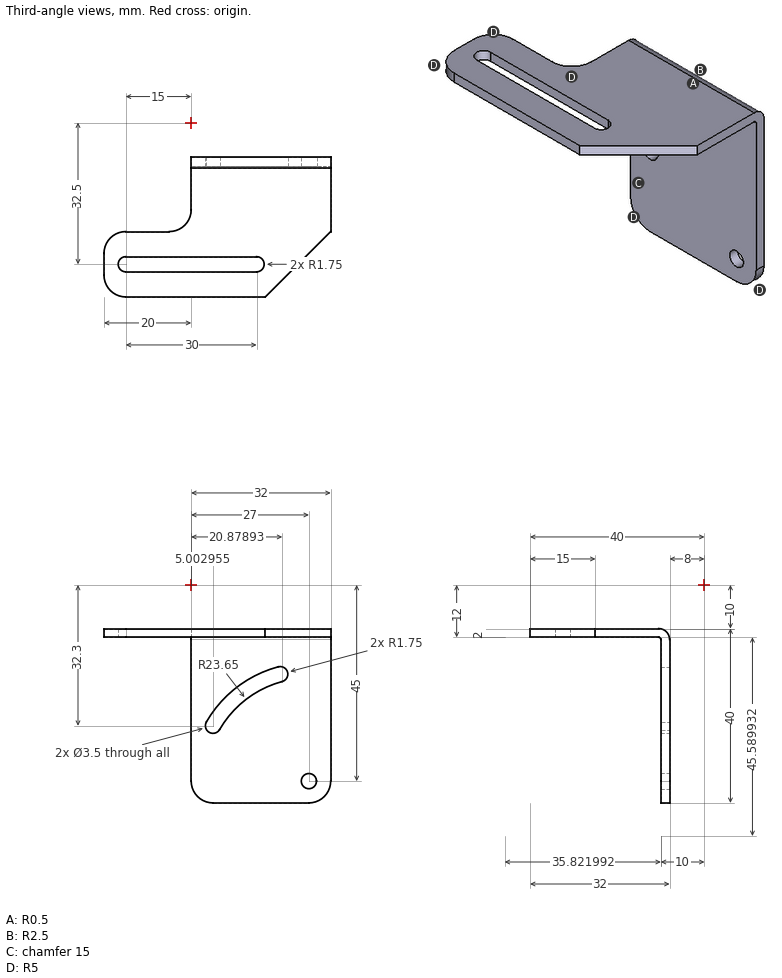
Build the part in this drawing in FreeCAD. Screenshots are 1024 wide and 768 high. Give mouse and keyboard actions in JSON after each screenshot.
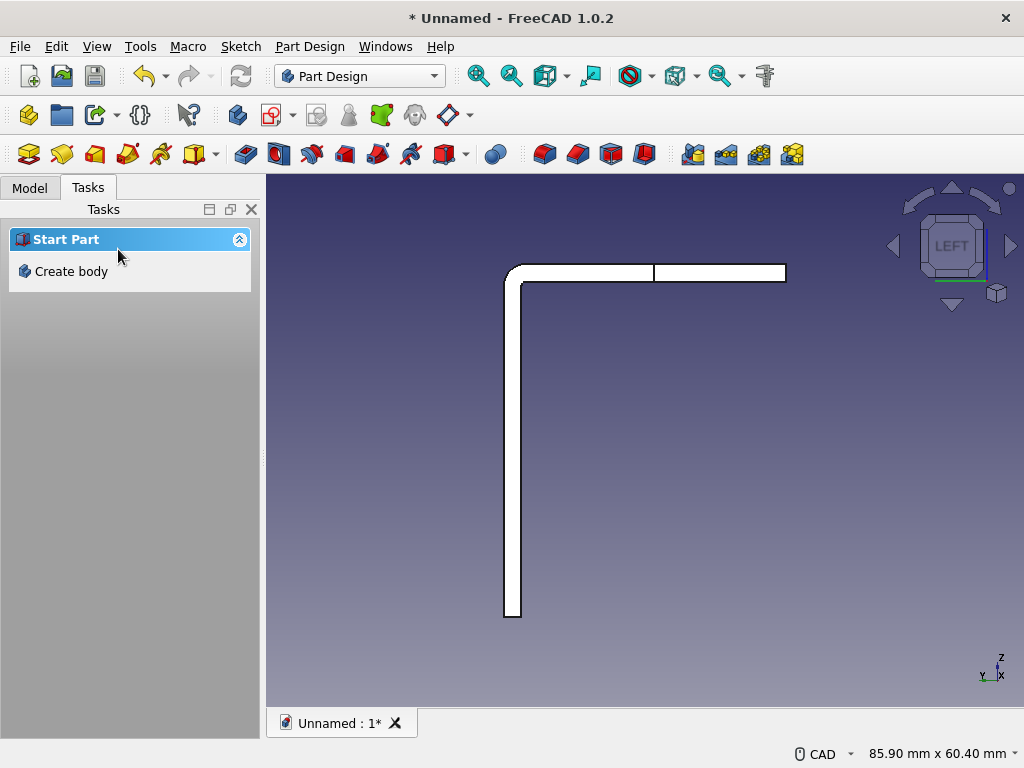
{"action": "key", "text": "5"}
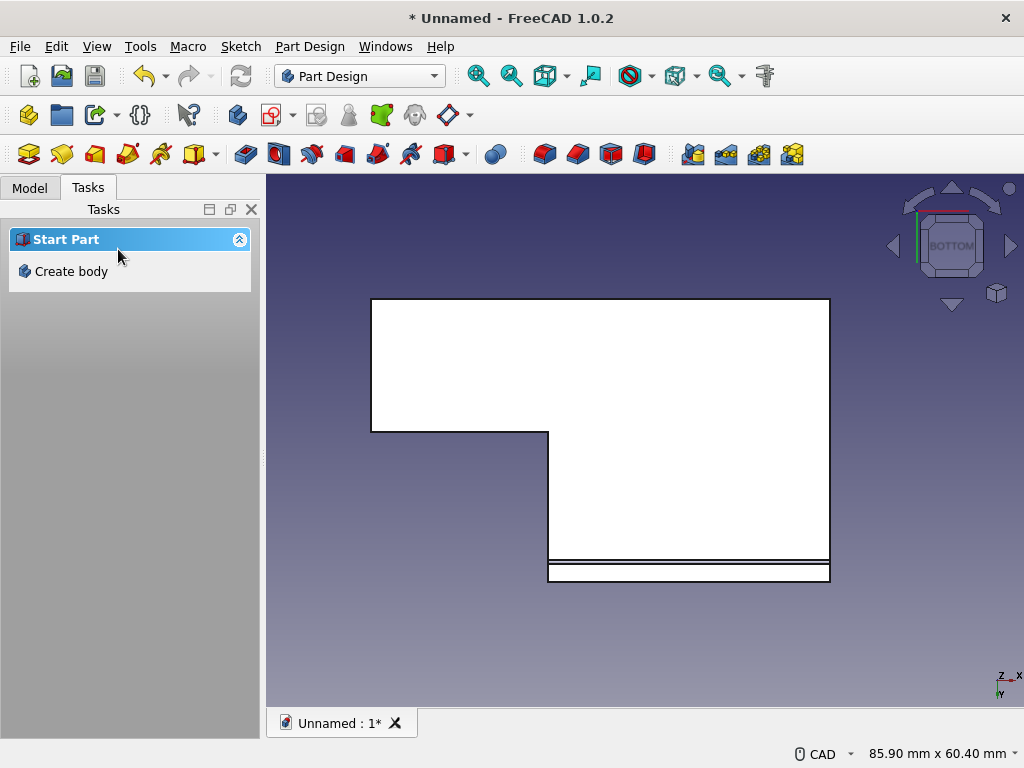
{"action": "left_click", "coordinate": [666, 428]}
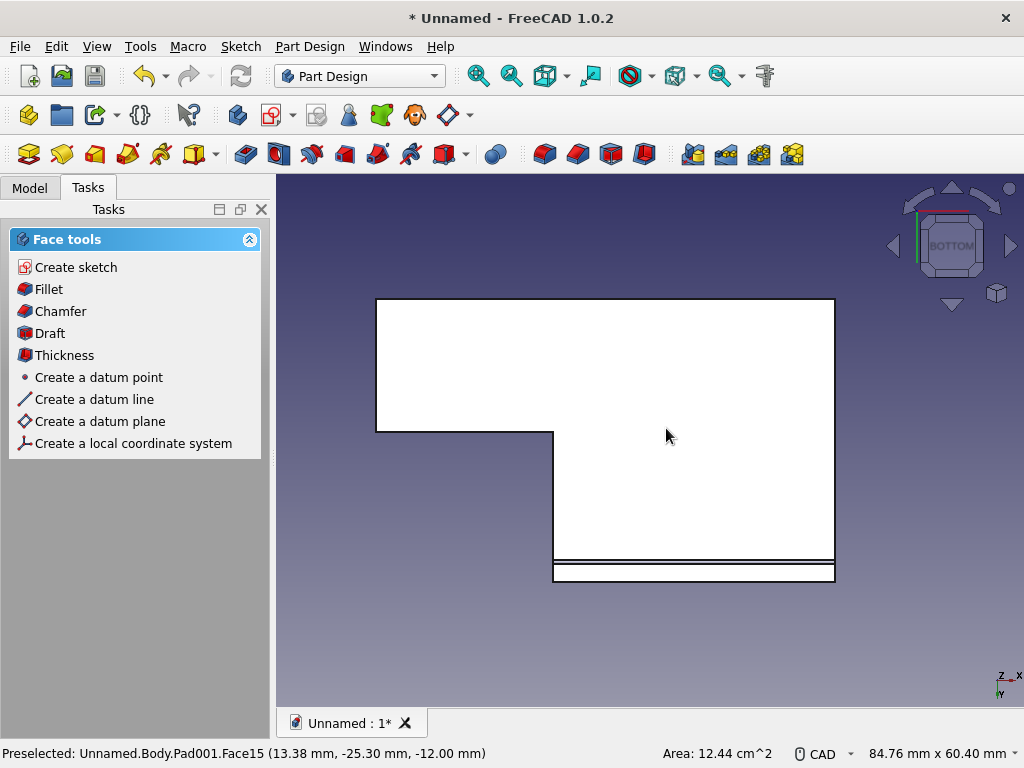
{"action": "left_click", "coordinate": [270, 116]}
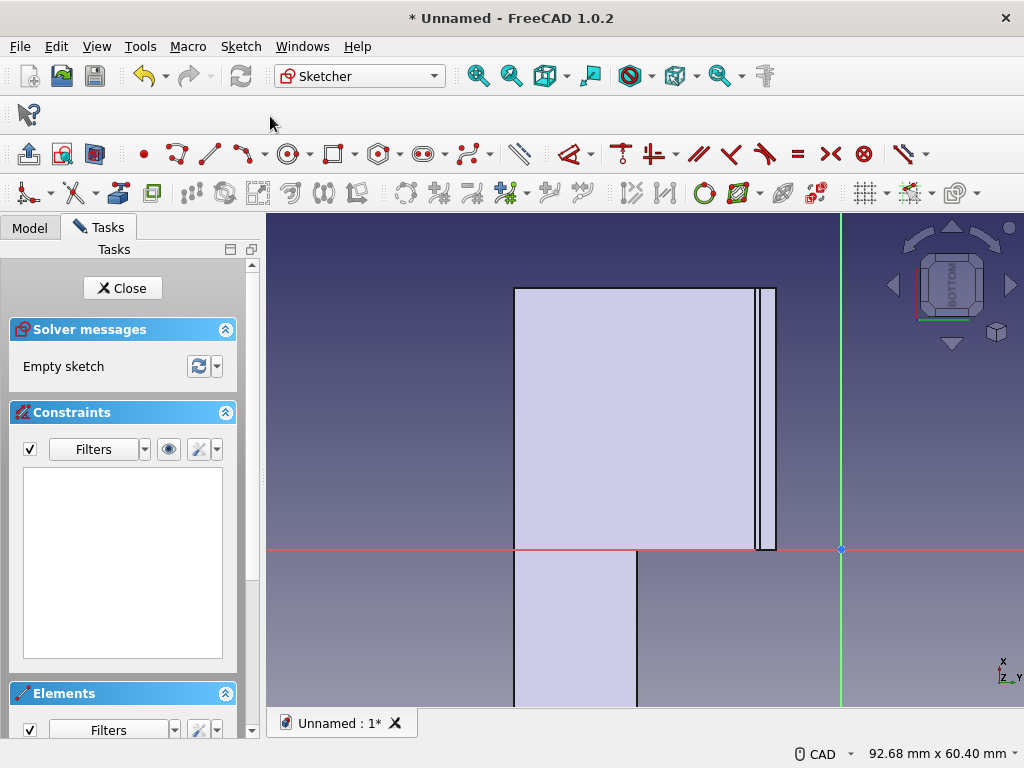
{"action": "scroll", "coordinate": [294, 241], "scroll_direction": "down", "scroll_amount": 1}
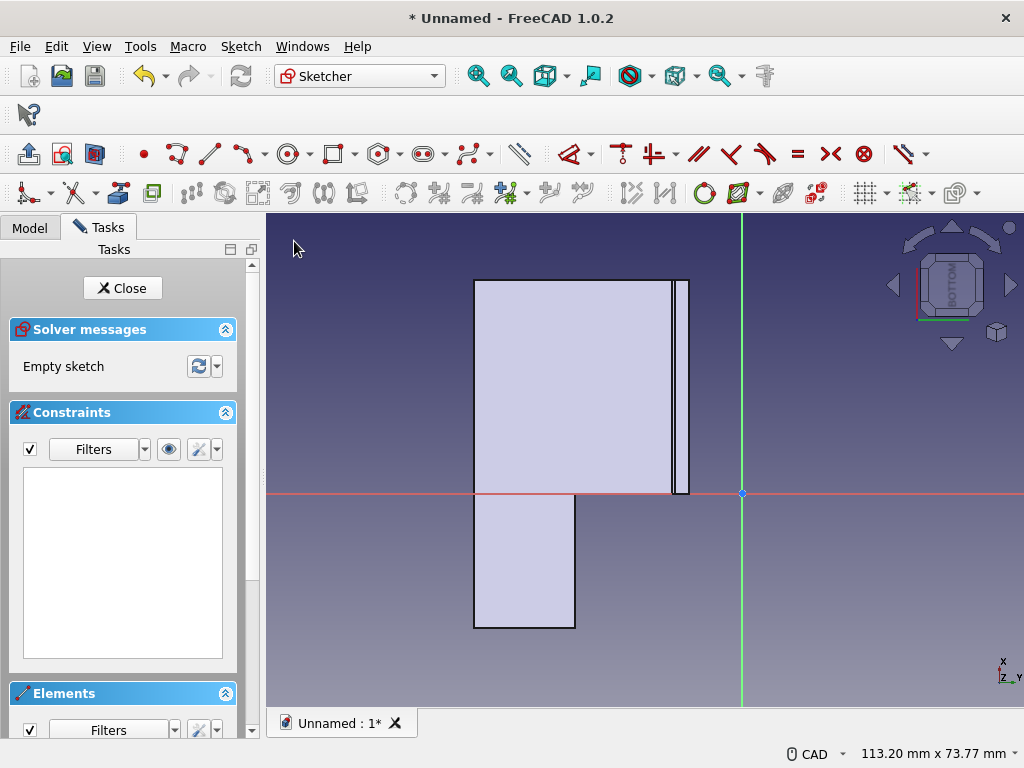
{"action": "scroll", "coordinate": [731, 563], "scroll_direction": "up", "scroll_amount": 2}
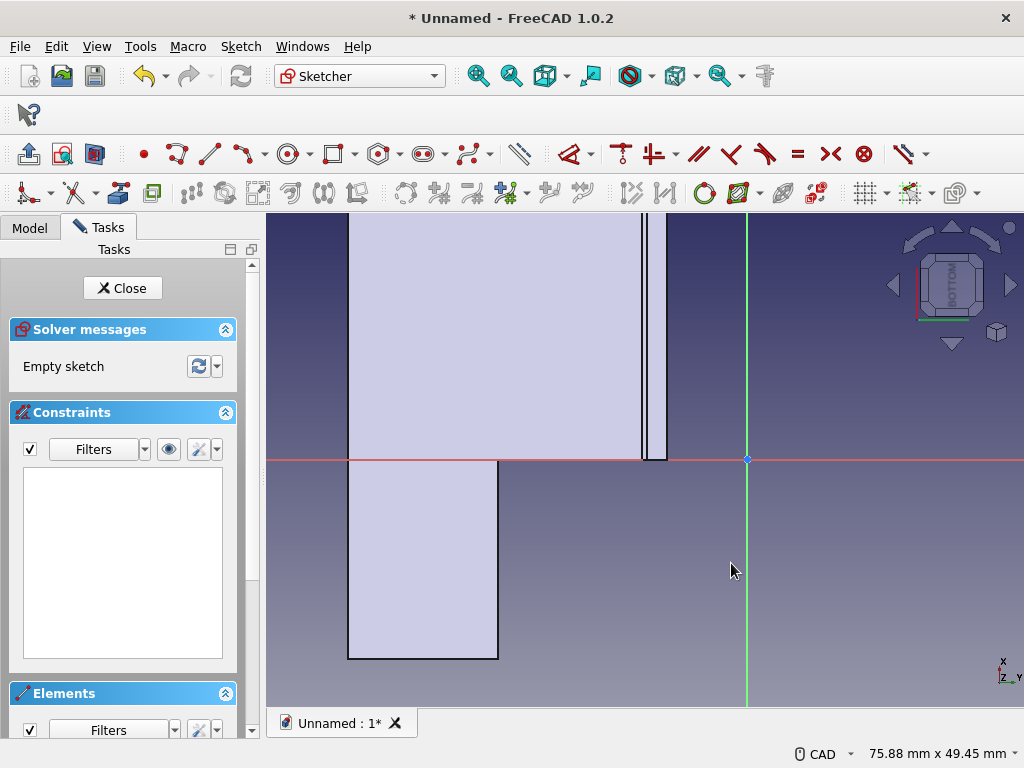
{"action": "key", "text": "g s"}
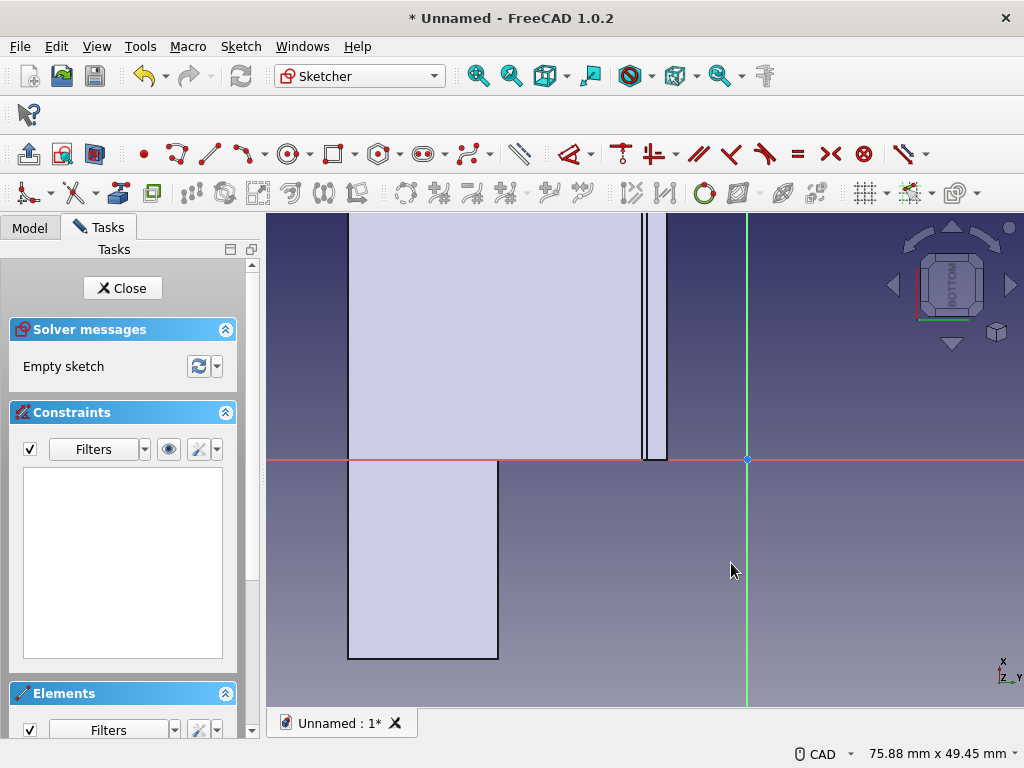
{"action": "scroll", "coordinate": [423, 610], "scroll_direction": "up", "scroll_amount": 2}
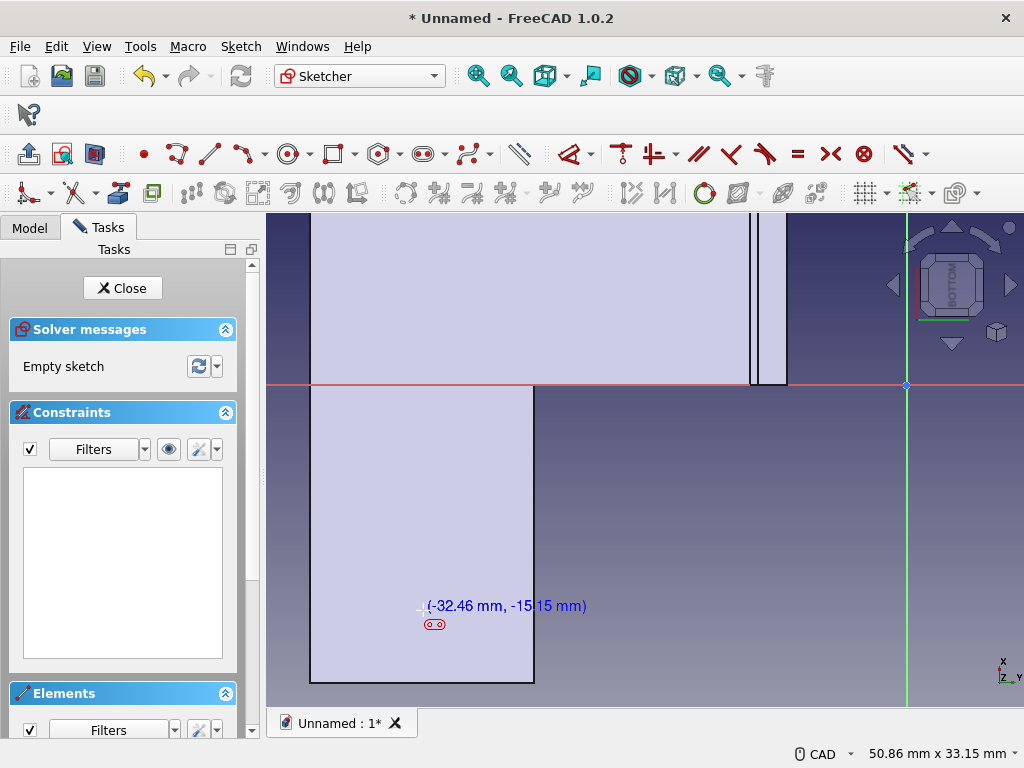
{"action": "left_click", "coordinate": [422, 609]}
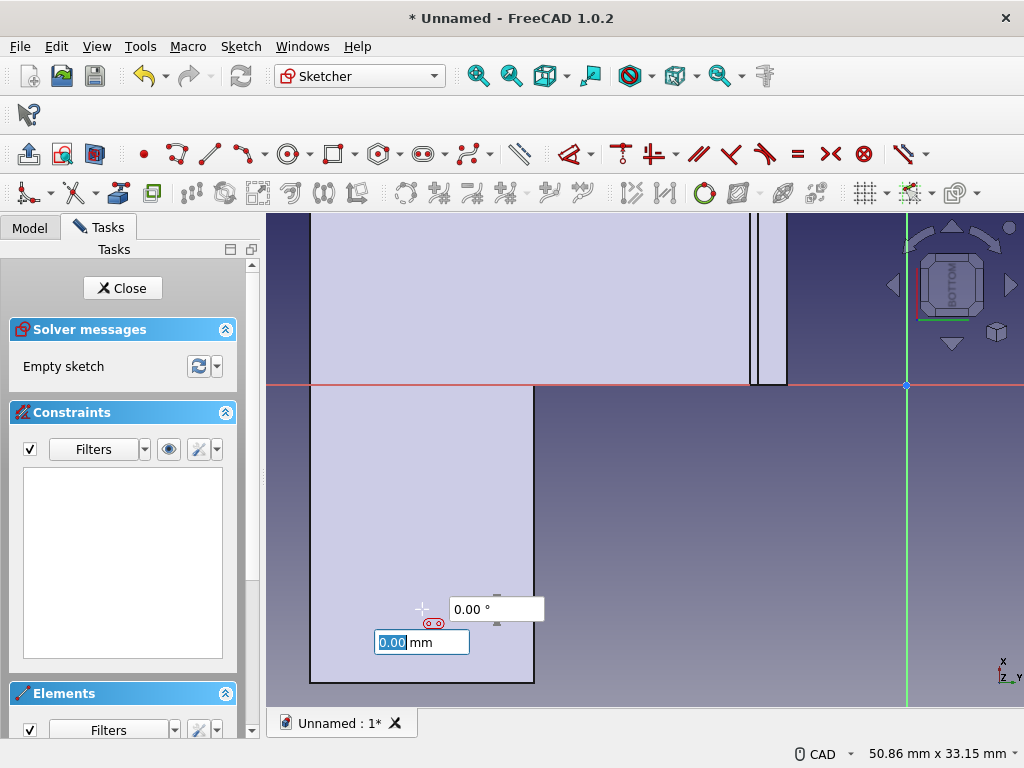
{"action": "scroll", "coordinate": [424, 612], "scroll_direction": "down", "scroll_amount": 2}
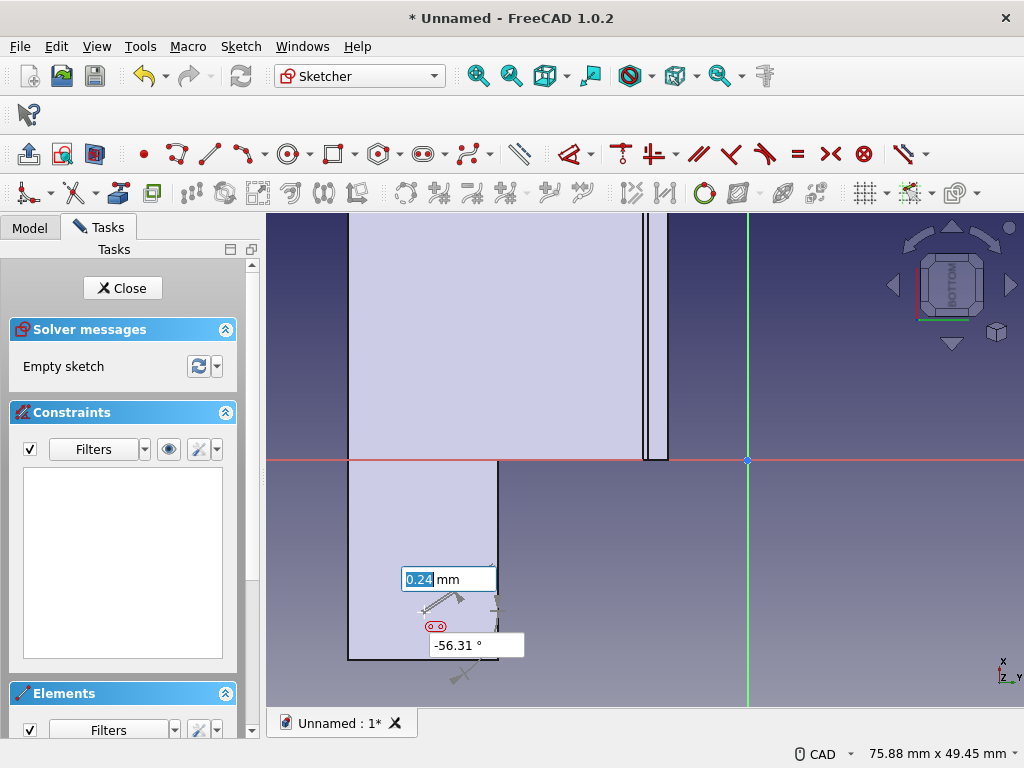
{"action": "left_click", "coordinate": [423, 310]}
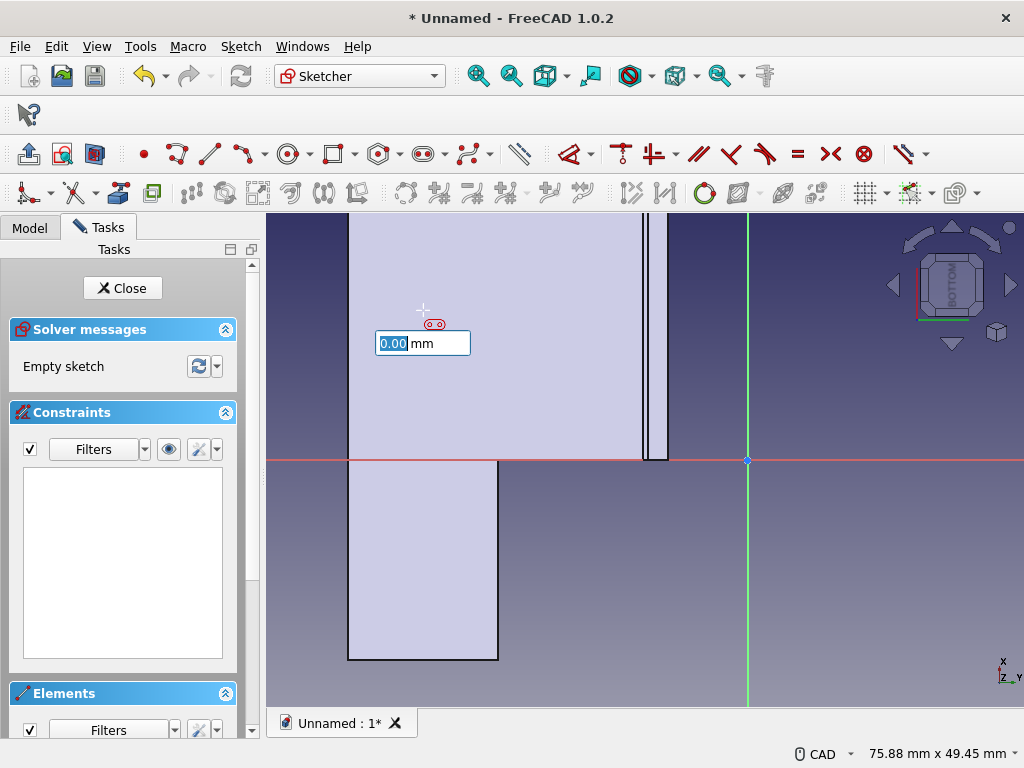
{"action": "left_click", "coordinate": [440, 505]}
{"action": "key", "text": "Escape"}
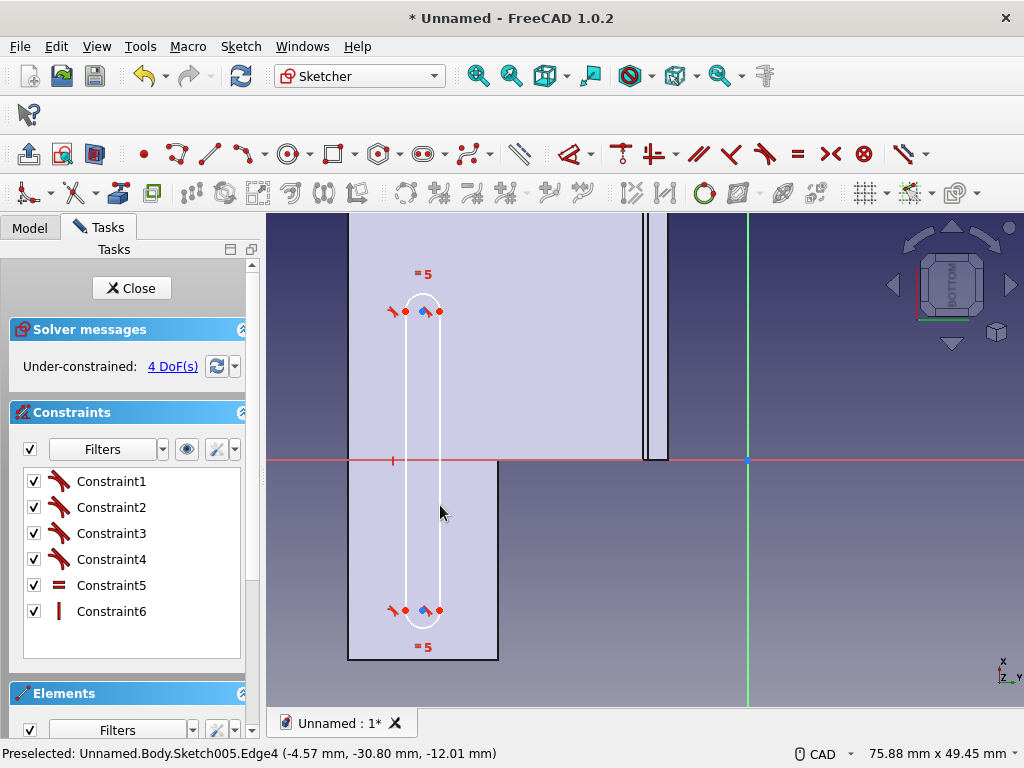
{"action": "key", "text": "d"}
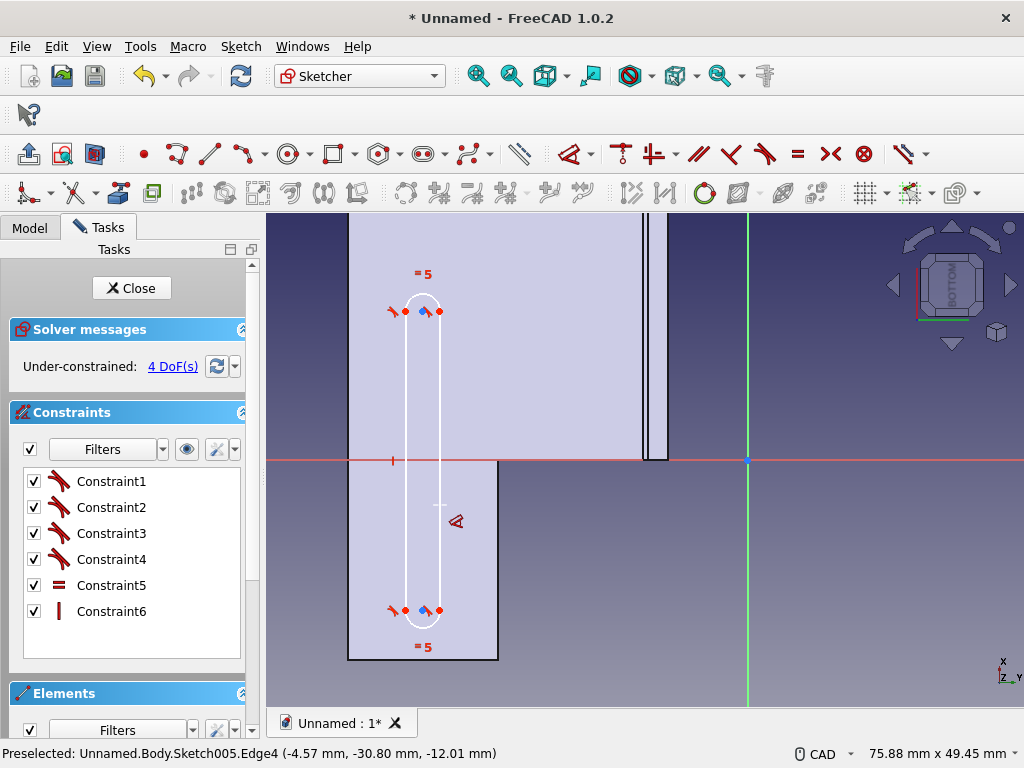
{"action": "scroll", "coordinate": [413, 625], "scroll_direction": "up", "scroll_amount": 5}